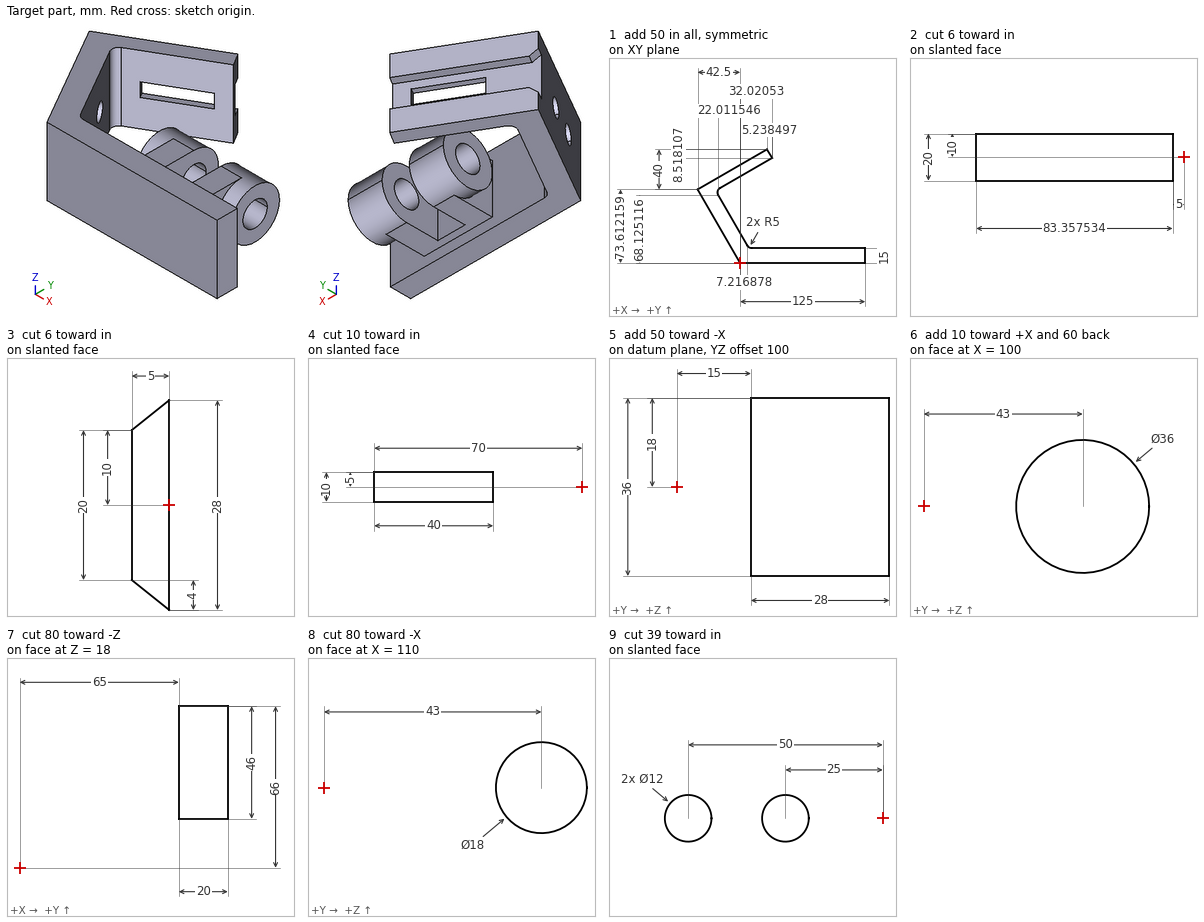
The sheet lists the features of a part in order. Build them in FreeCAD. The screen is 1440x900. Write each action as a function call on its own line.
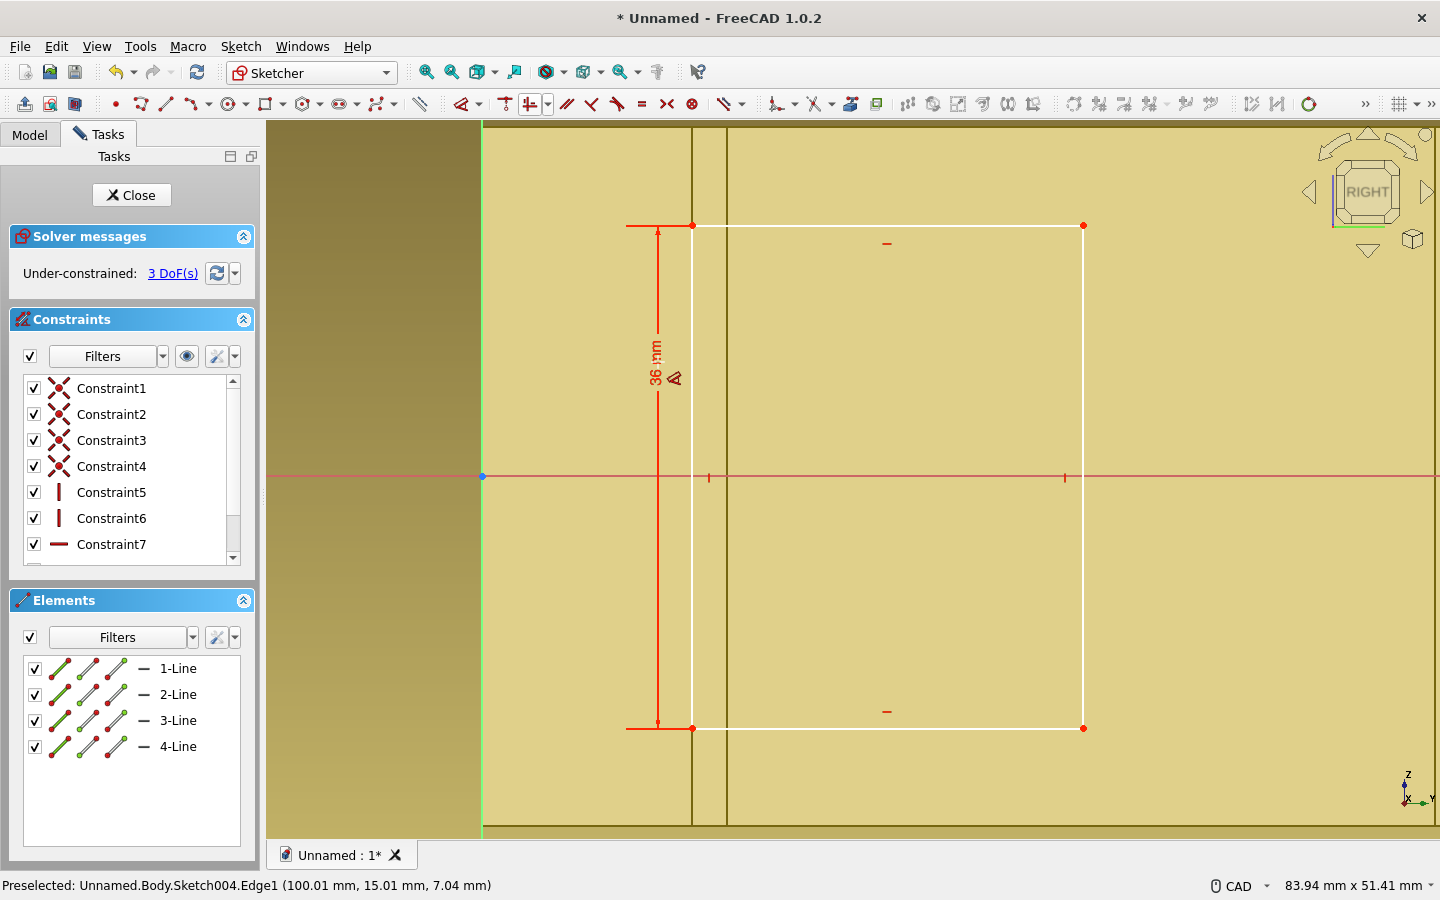
click(809, 729)
click(887, 763)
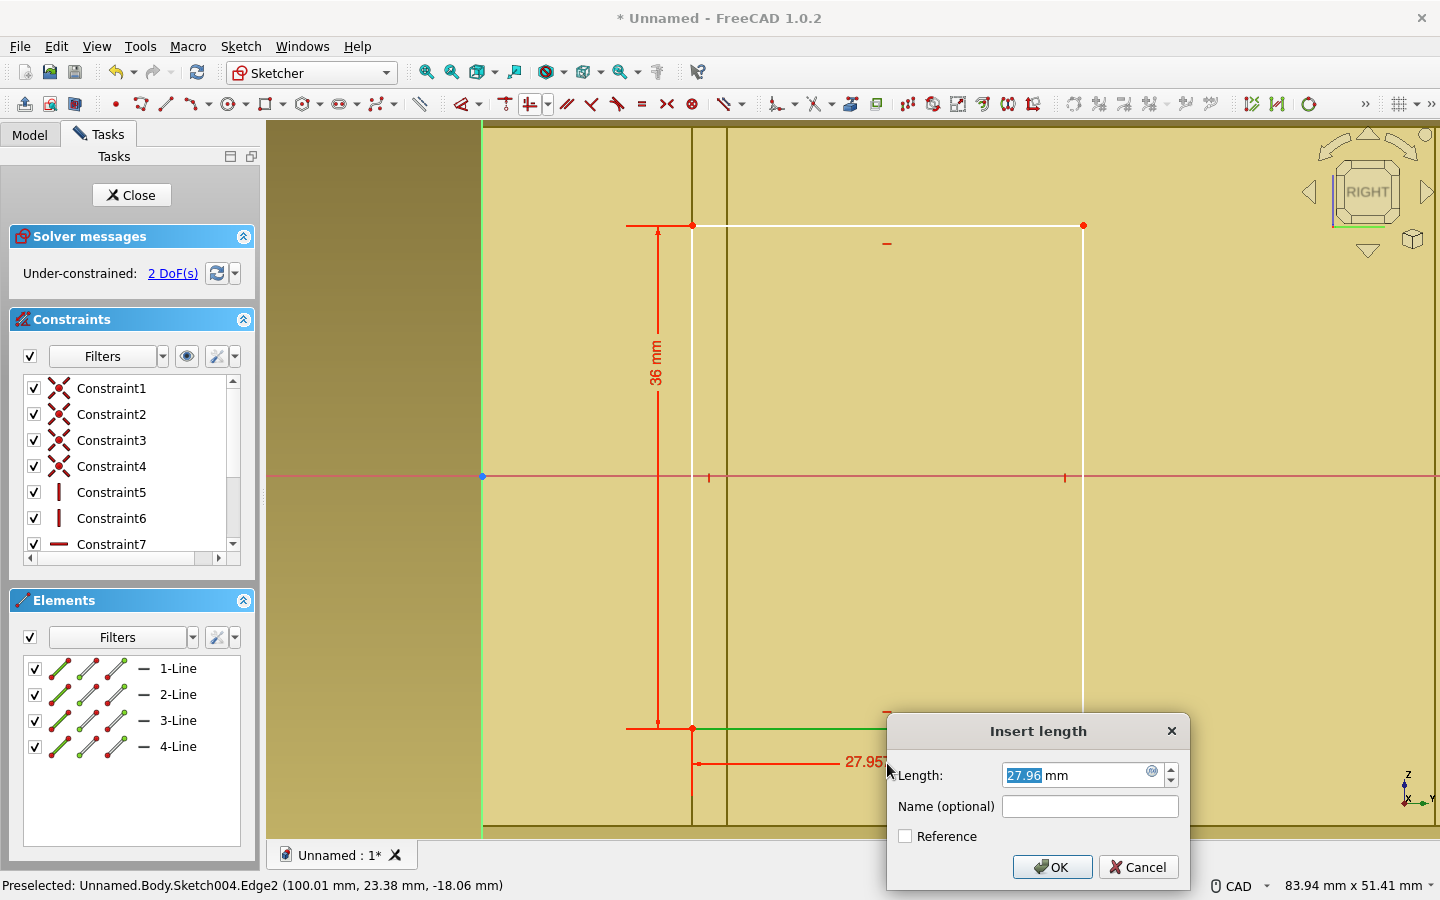
text(28)
key(Return)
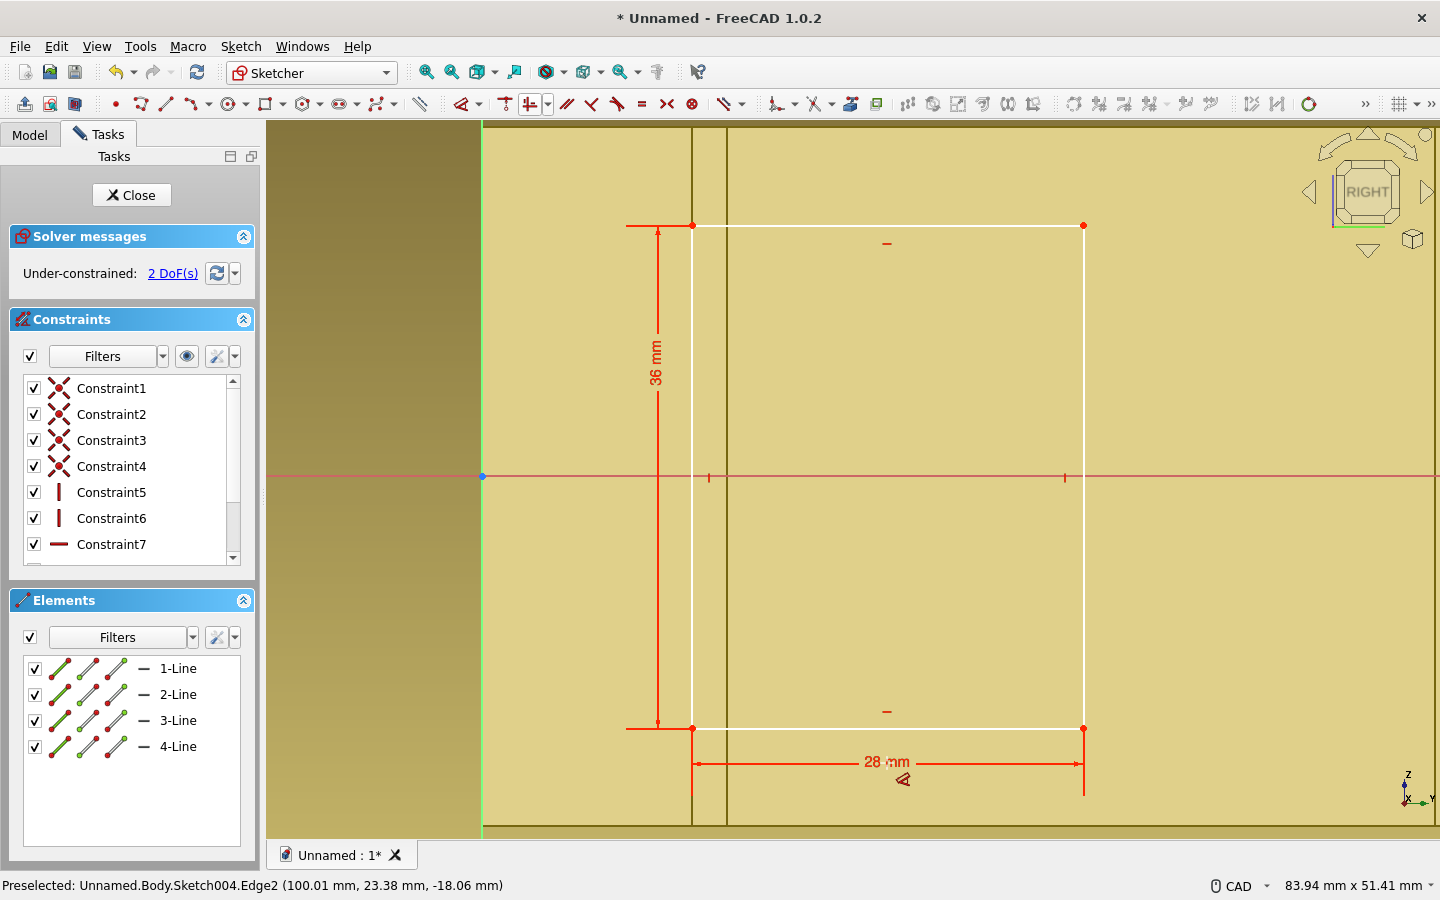
click(692, 226)
click(587, 192)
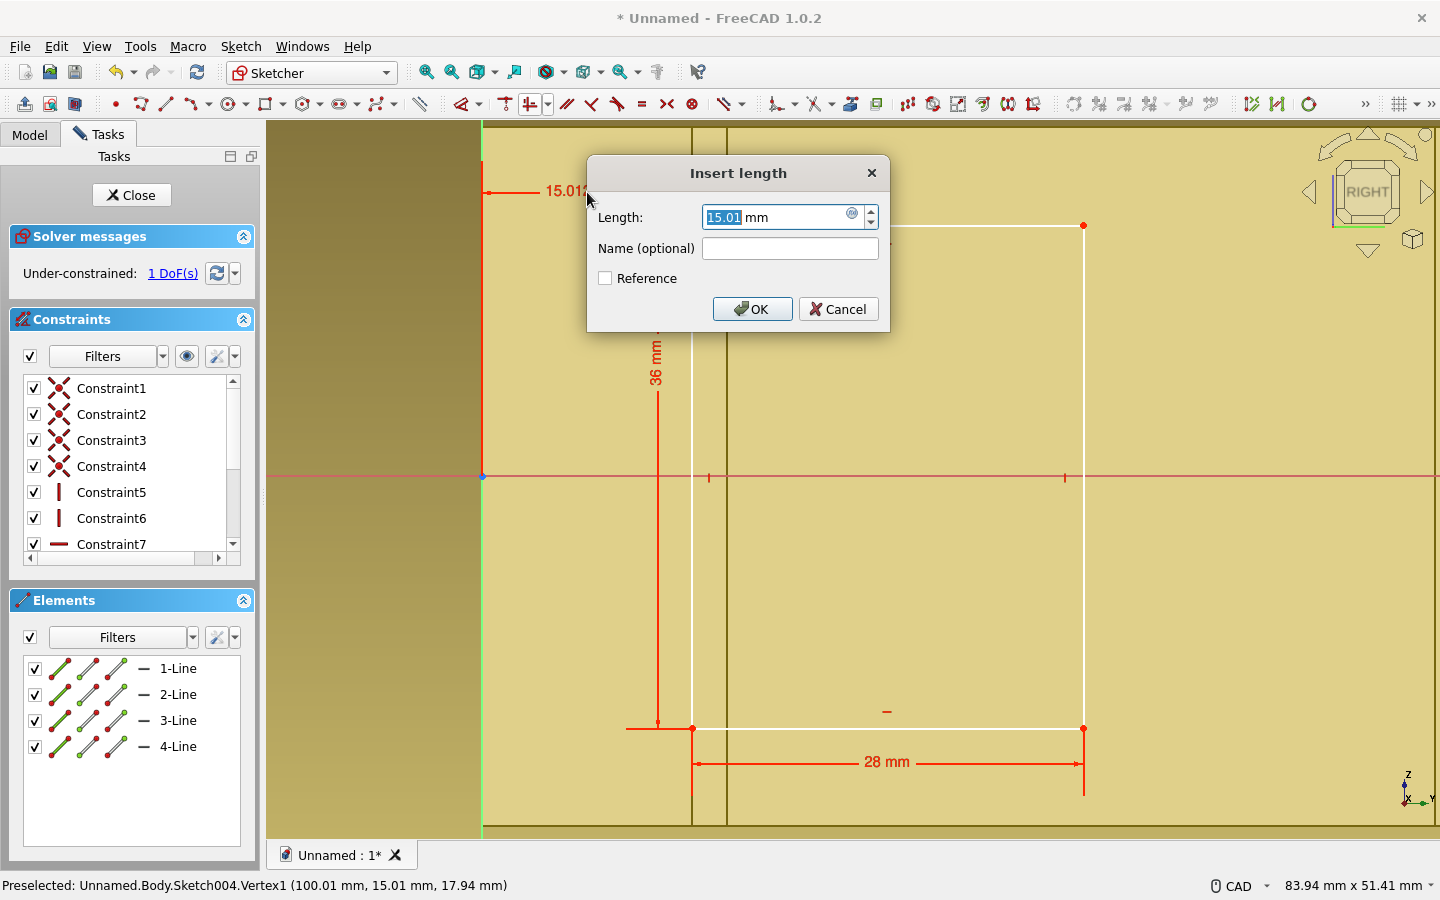
text(15)
key(Return)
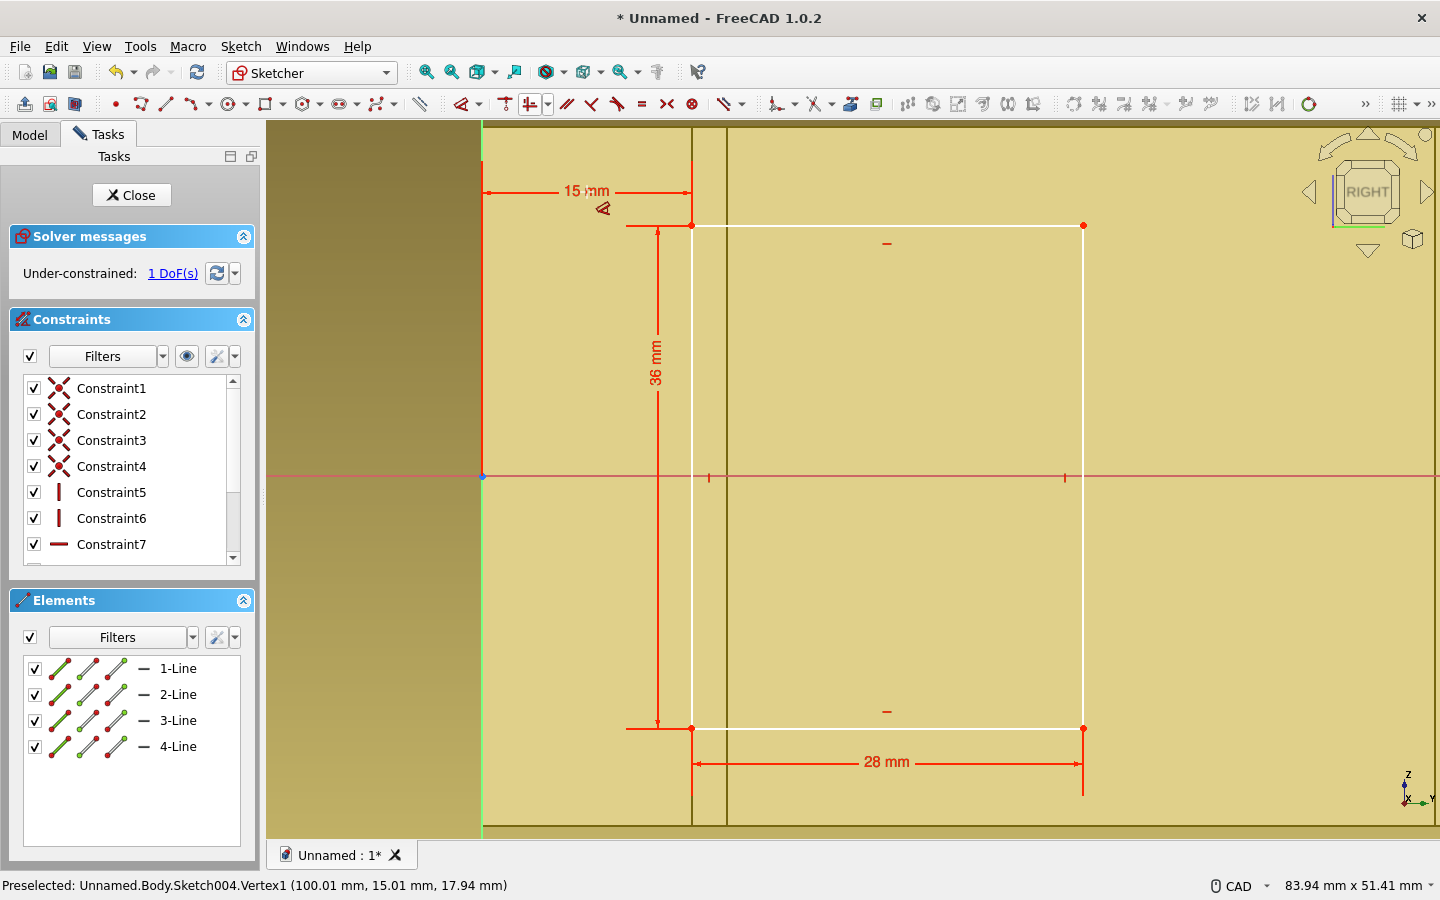
click(692, 226)
click(448, 351)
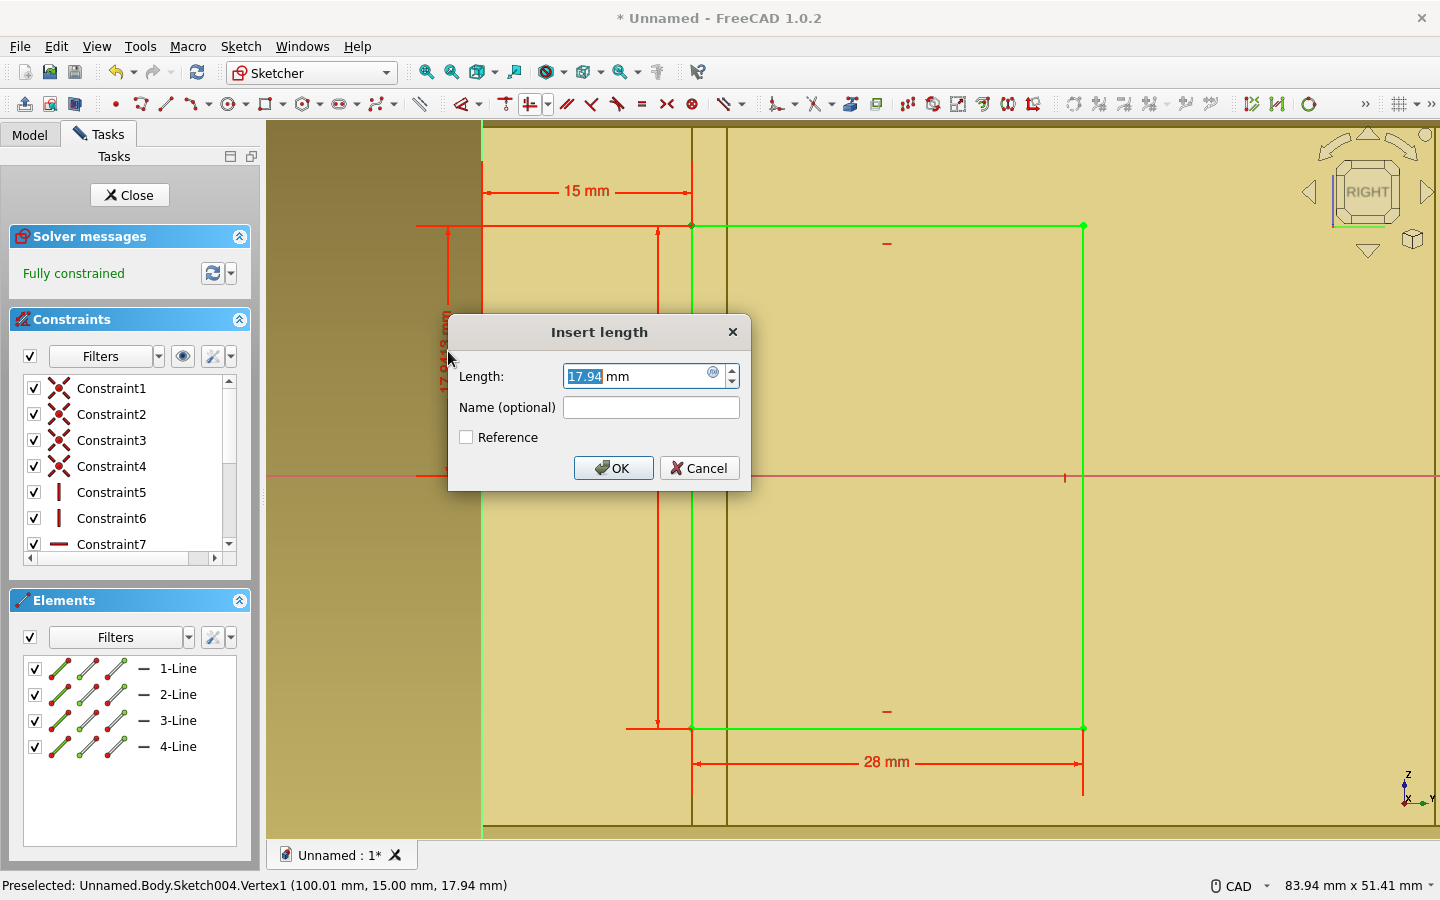
text(18)
key(Return)
key(Escape)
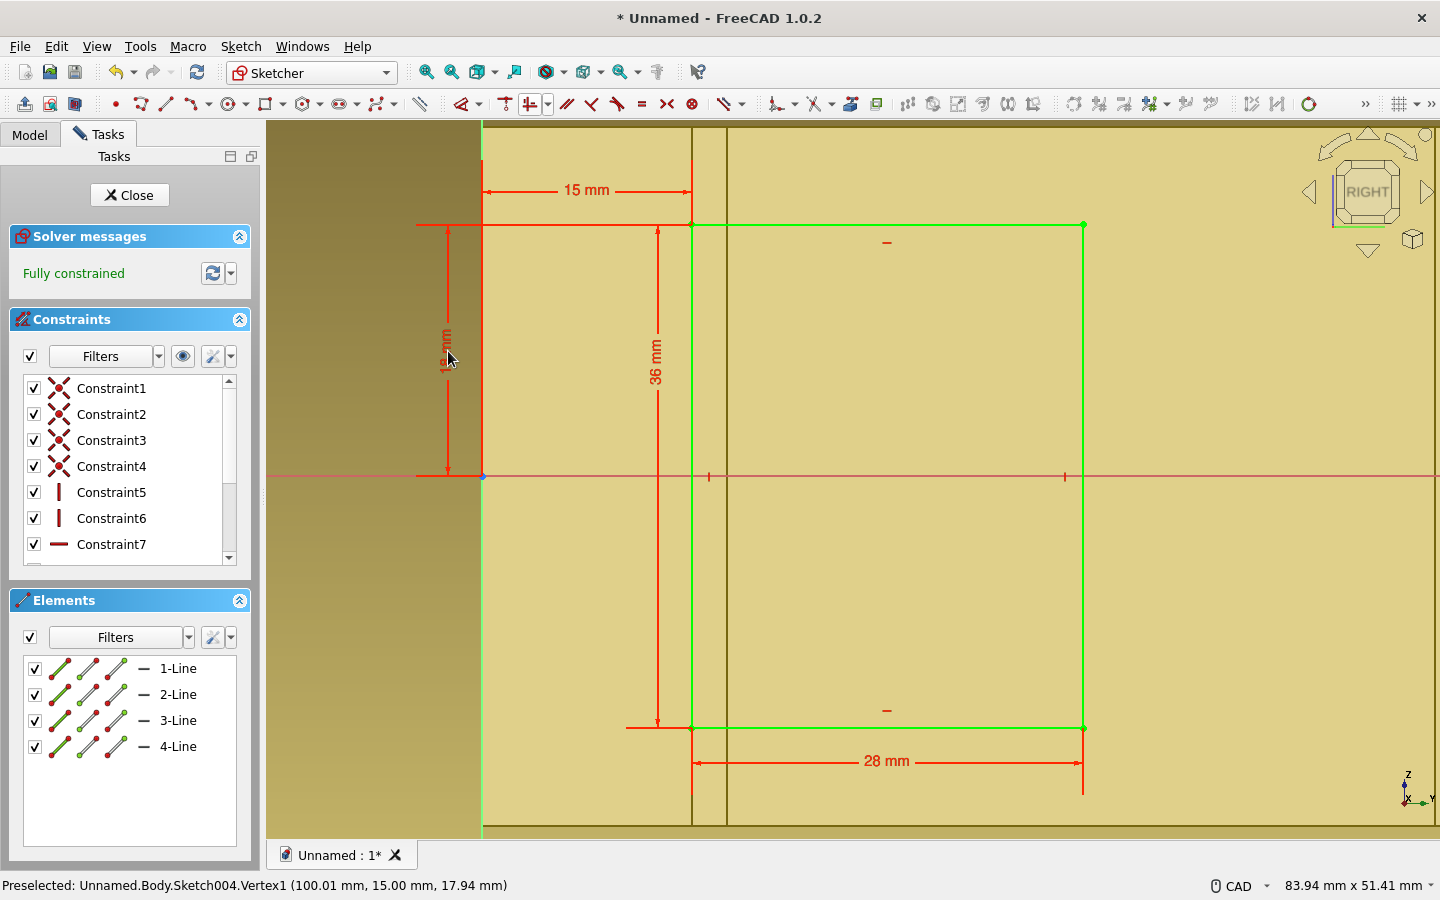
click(130, 195)